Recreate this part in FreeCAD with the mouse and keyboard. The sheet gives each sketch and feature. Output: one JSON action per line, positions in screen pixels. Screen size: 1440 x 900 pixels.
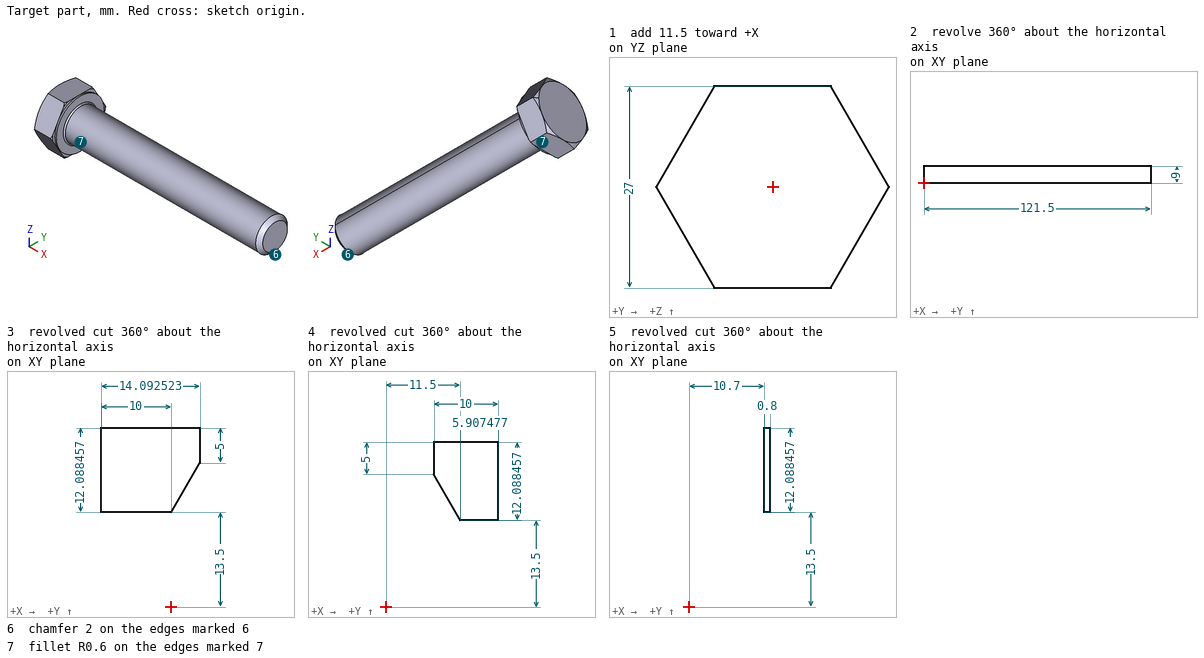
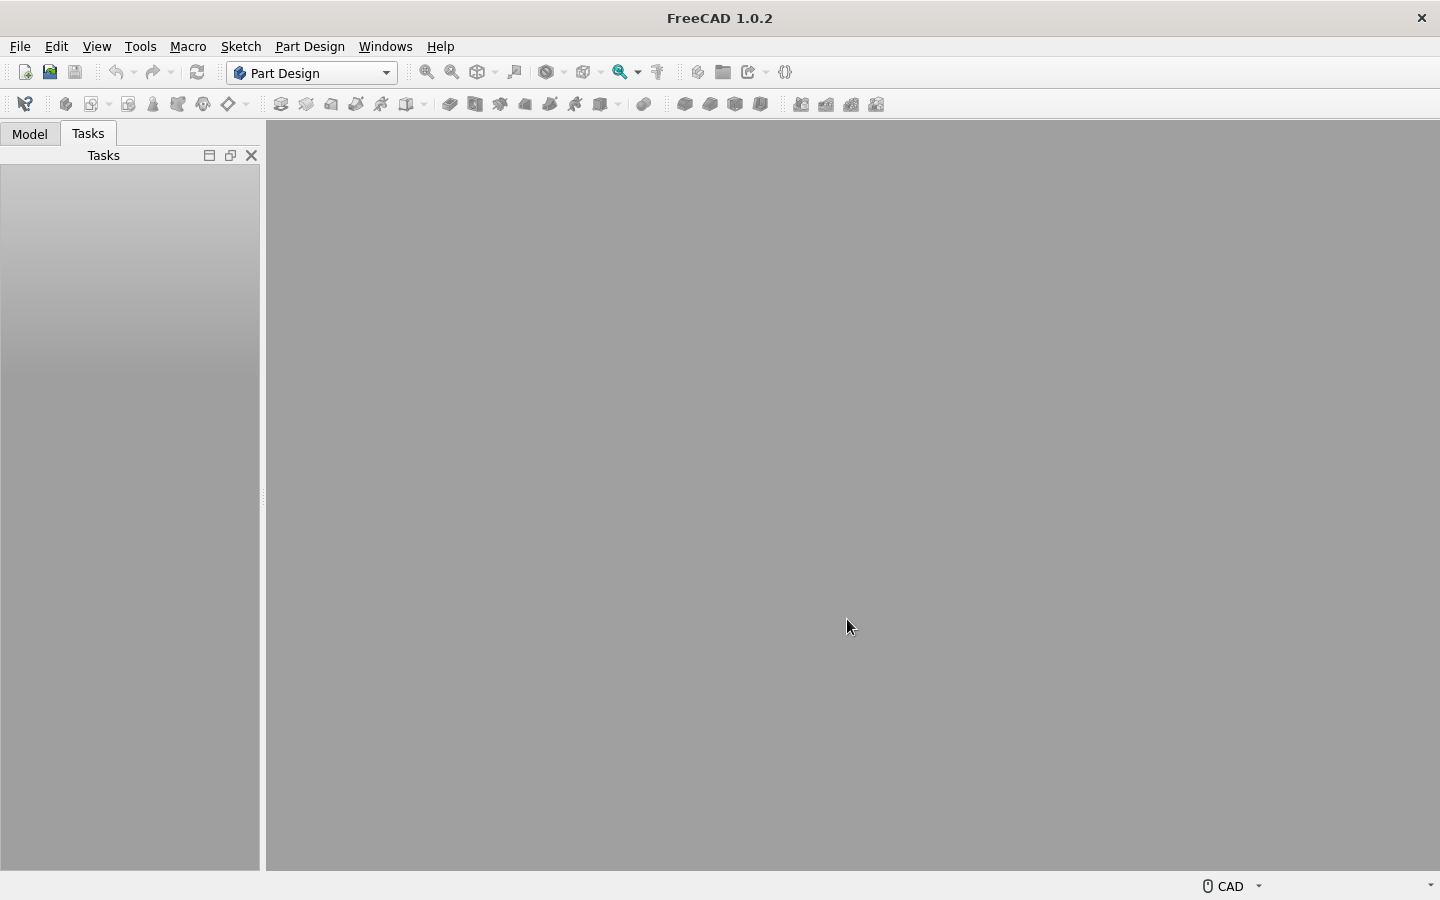
{"action": "left_click", "coordinate": [25, 72]}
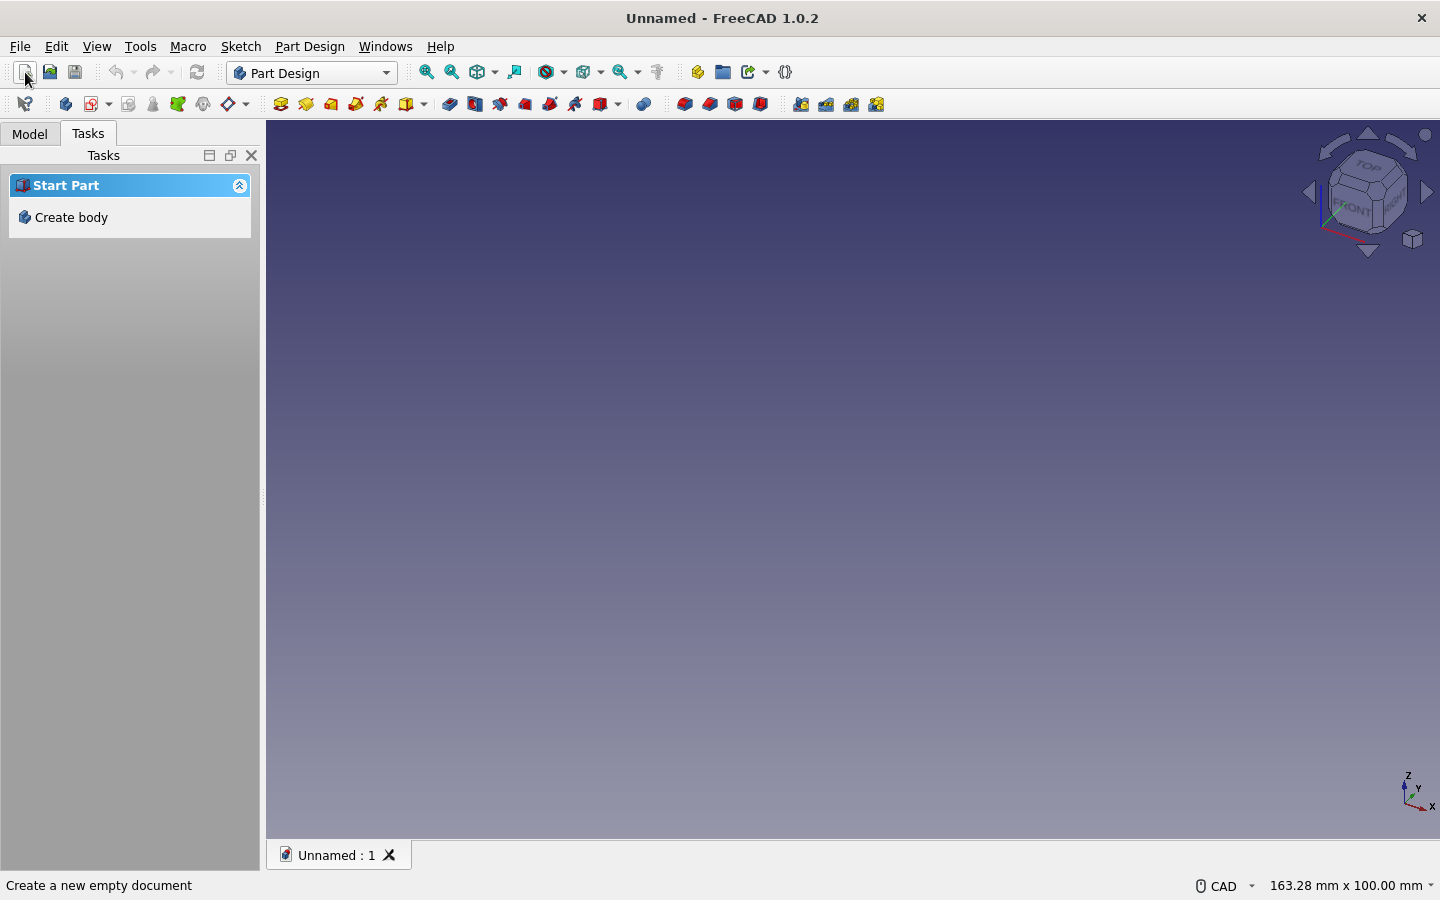
{"action": "left_click", "coordinate": [90, 104]}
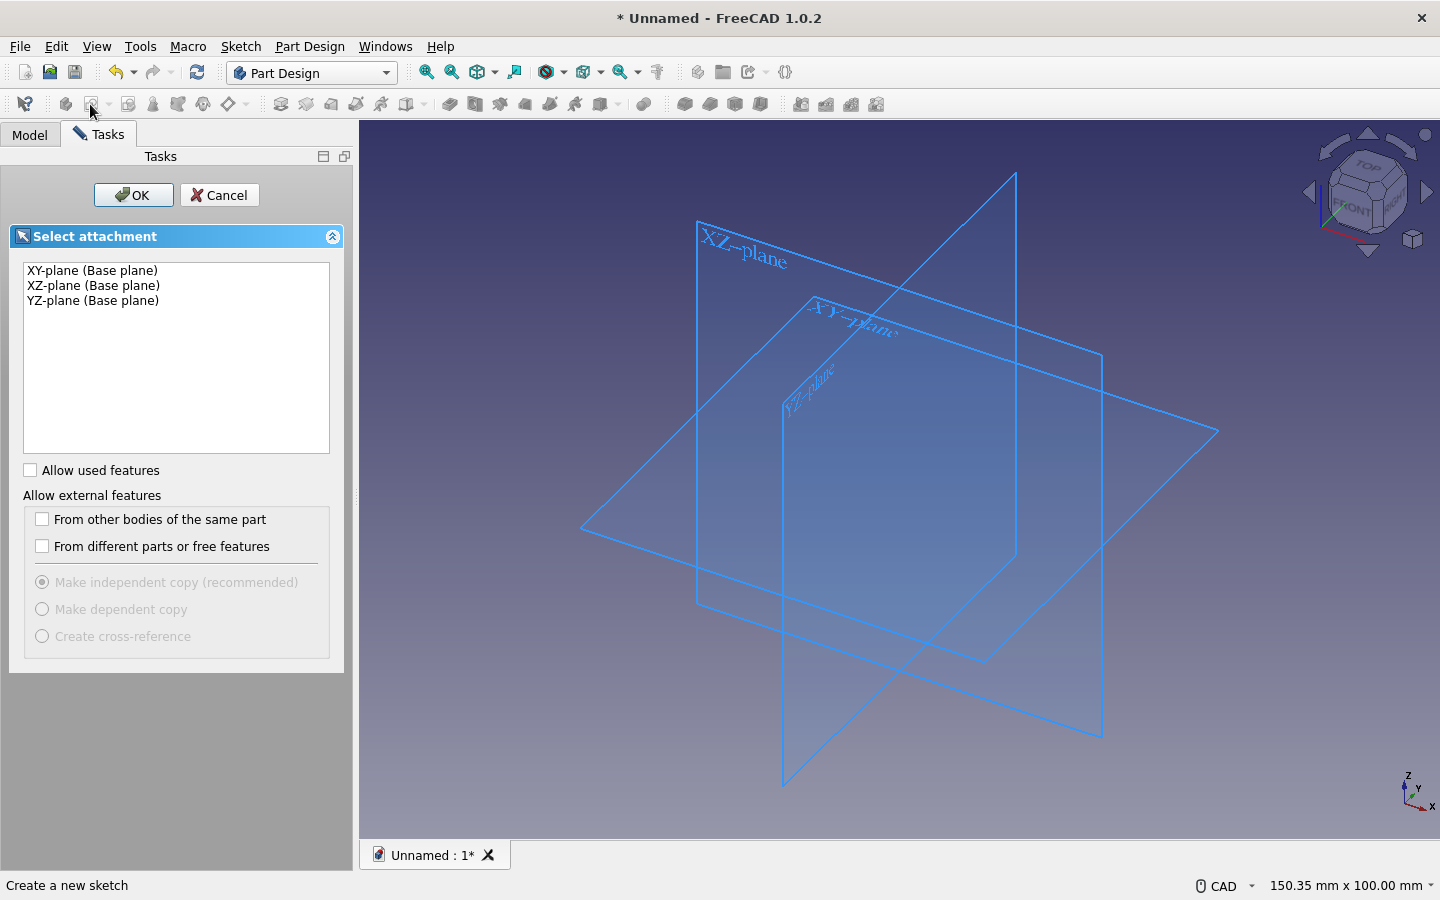
{"action": "left_click", "coordinate": [84, 300]}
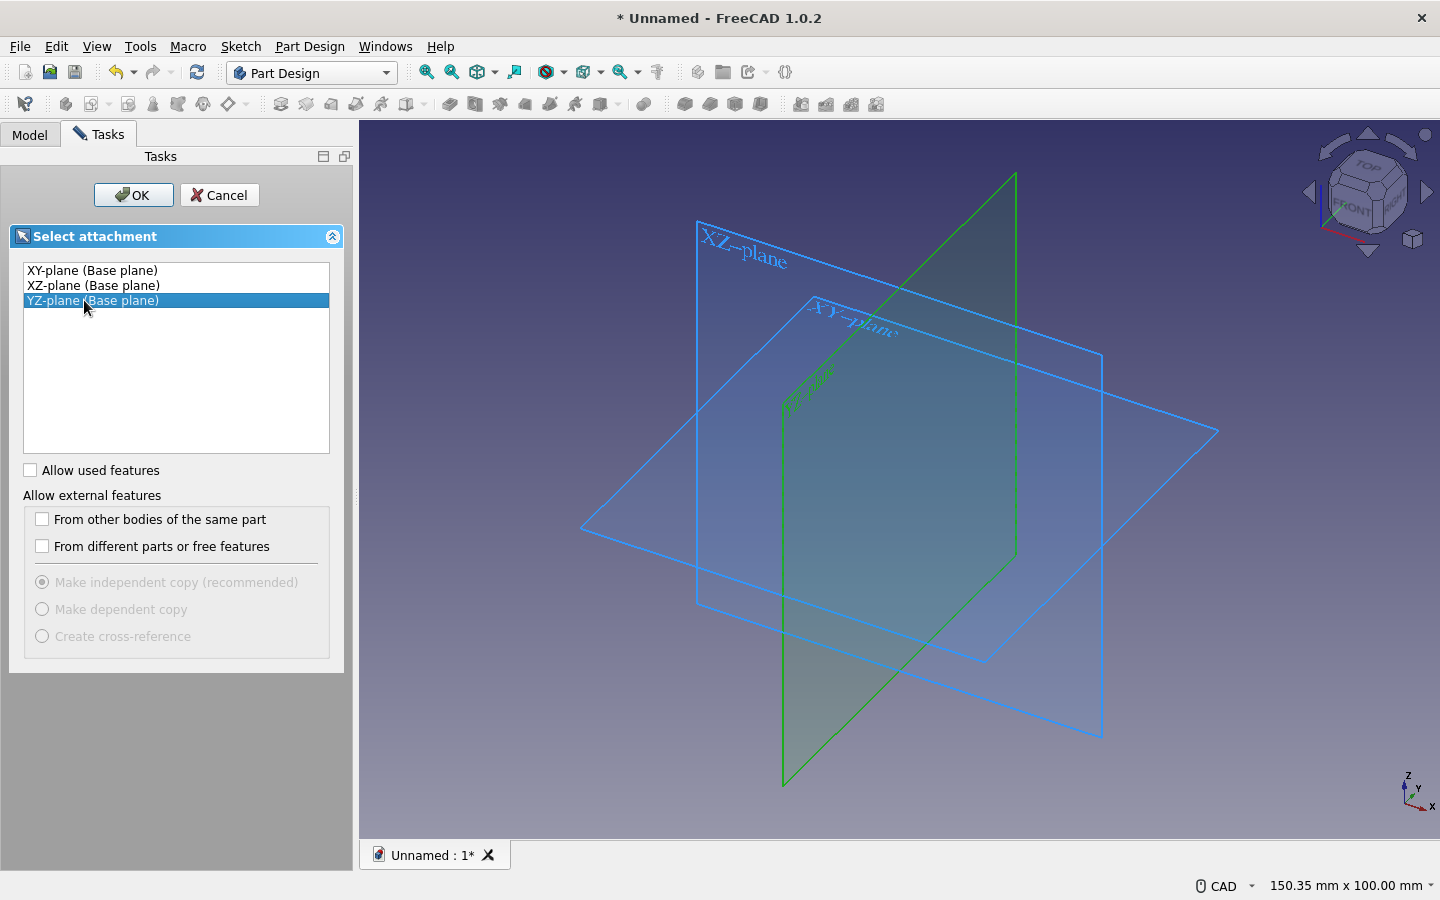
{"action": "left_click", "coordinate": [134, 195]}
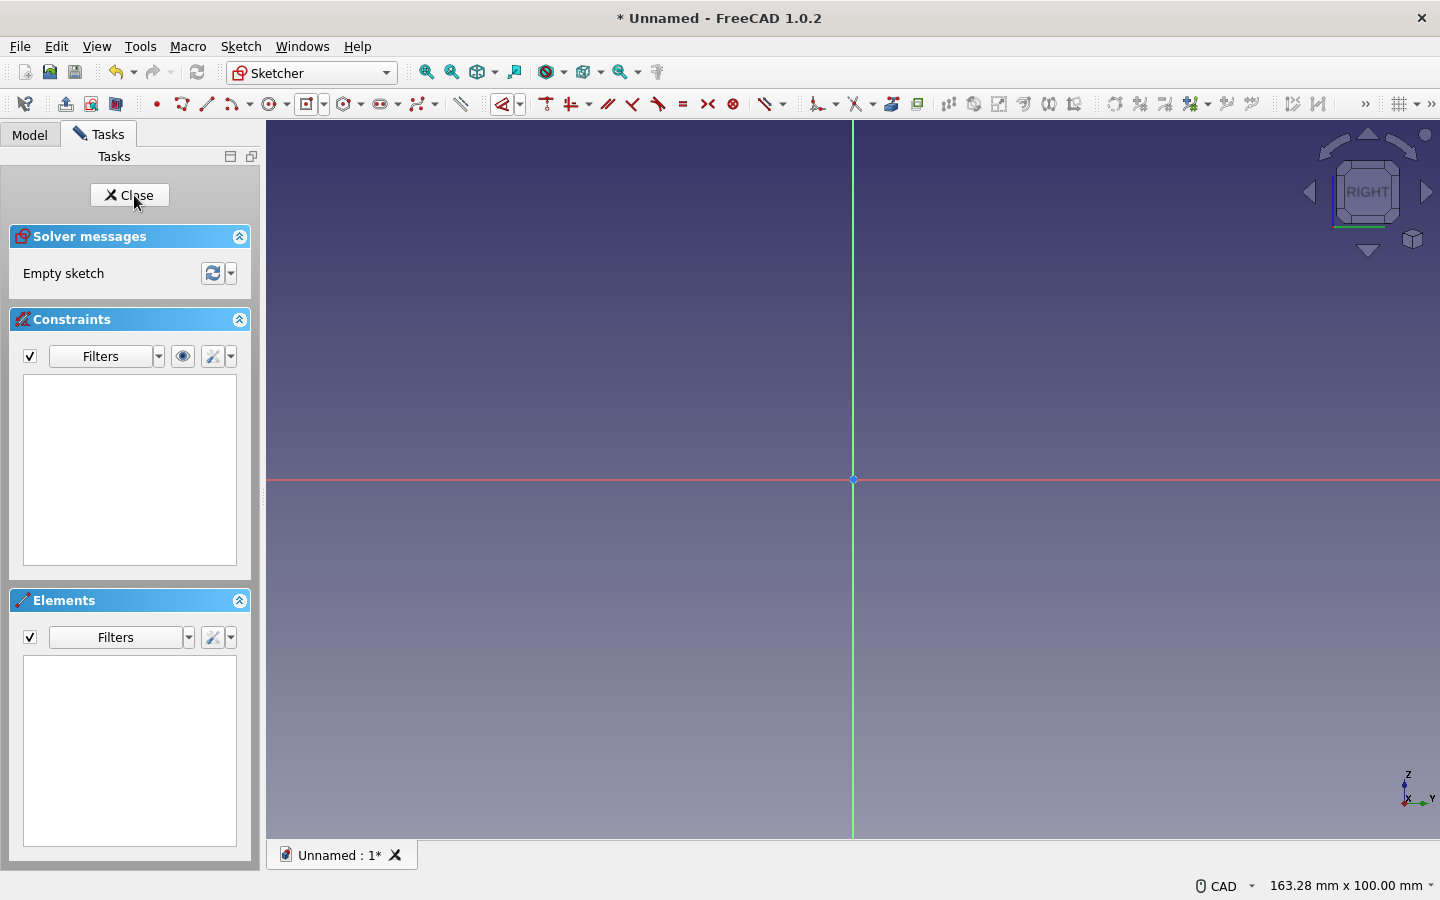
{"action": "scroll", "coordinate": [909, 480], "scroll_direction": "up", "scroll_amount": 4}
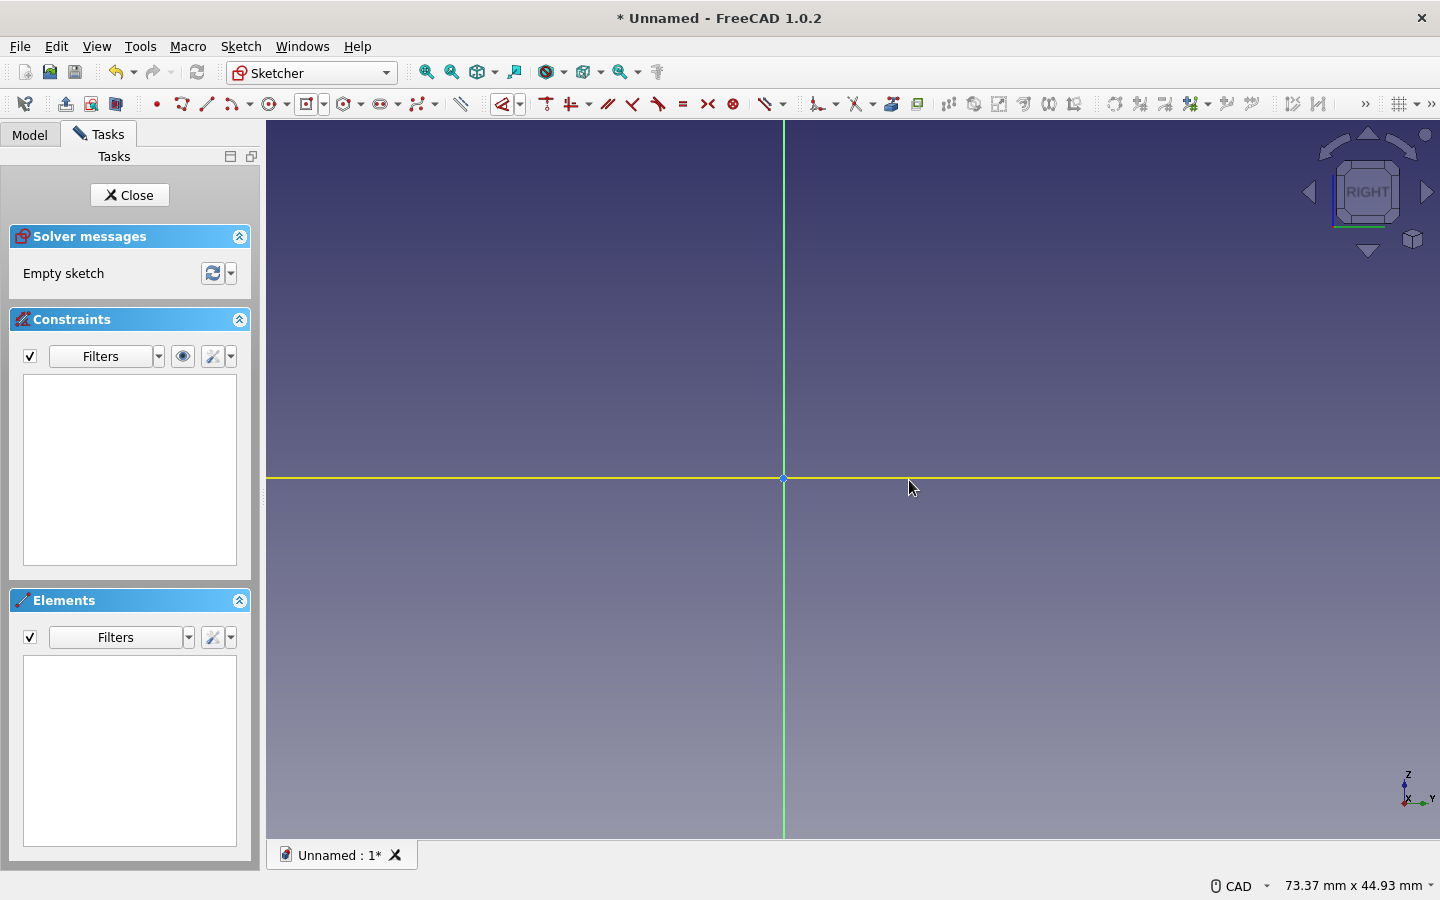
{"action": "left_click", "coordinate": [342, 104]}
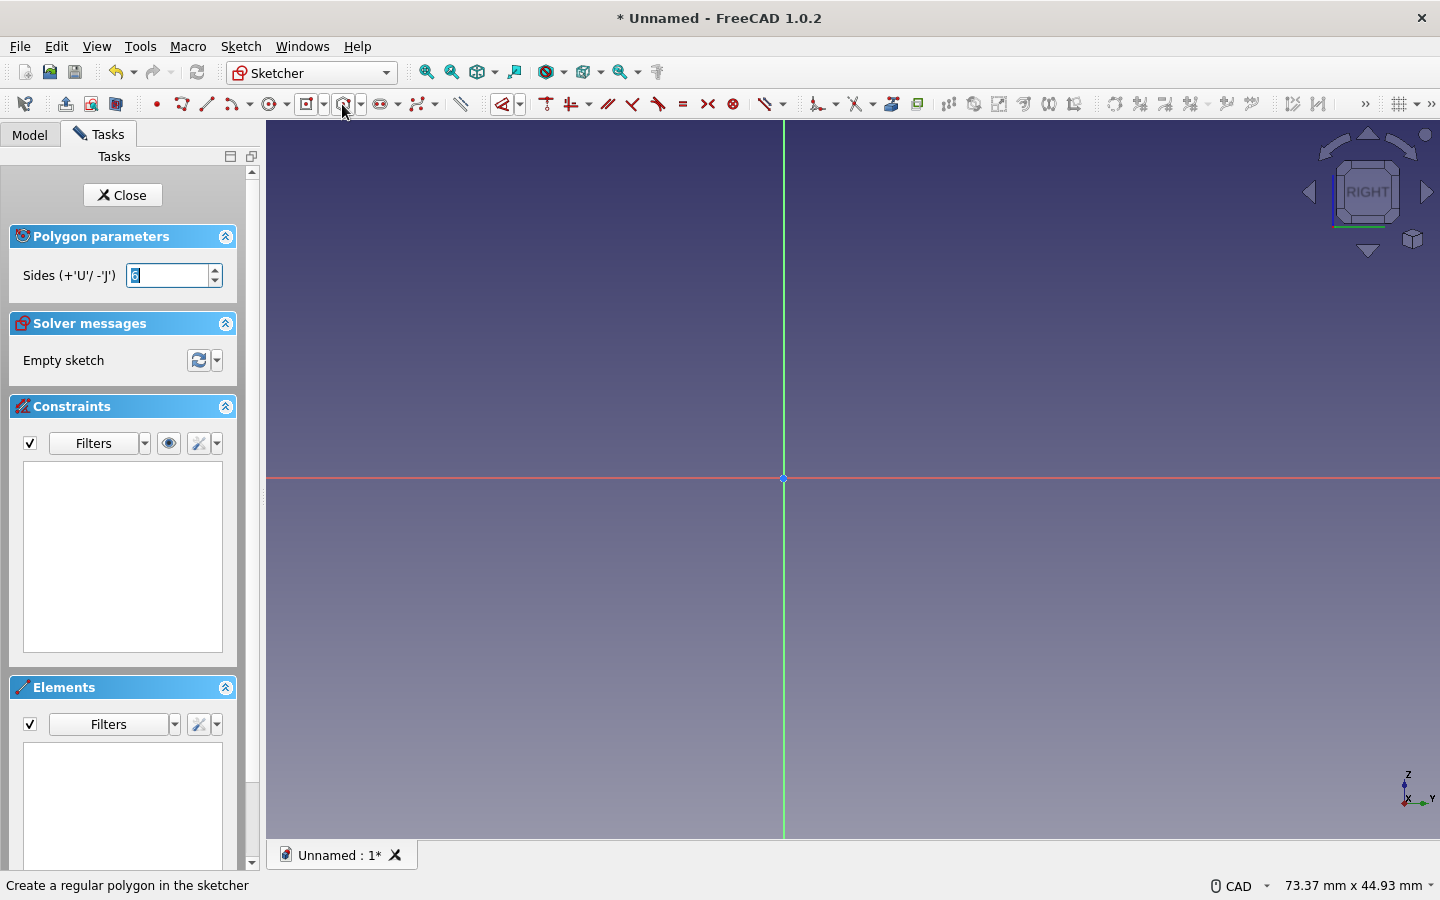
{"action": "left_click", "coordinate": [784, 478]}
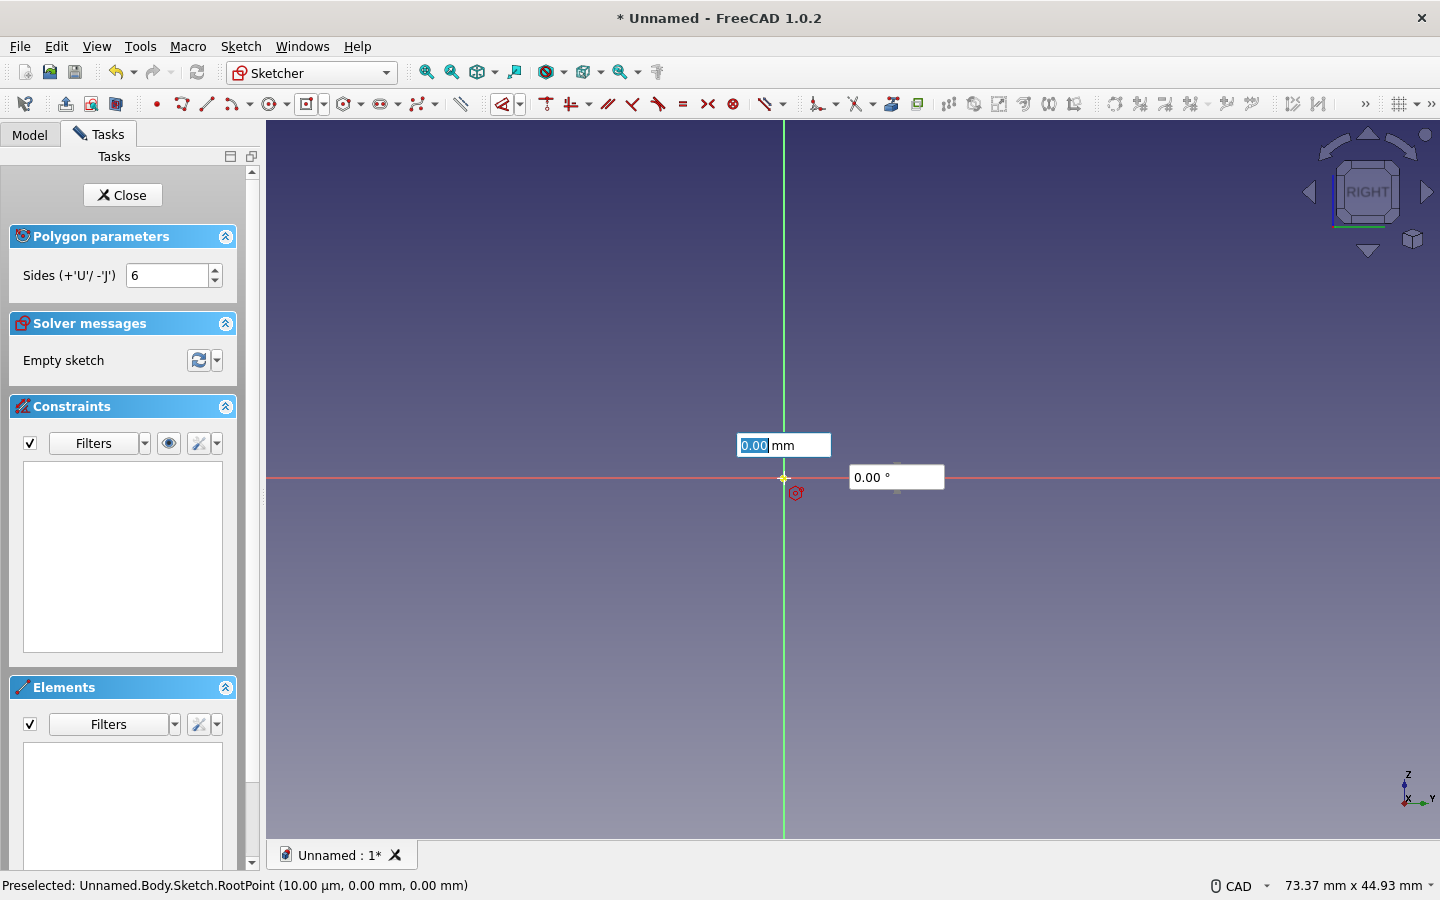
{"action": "left_click", "coordinate": [1033, 478]}
{"action": "key", "text": "Escape"}